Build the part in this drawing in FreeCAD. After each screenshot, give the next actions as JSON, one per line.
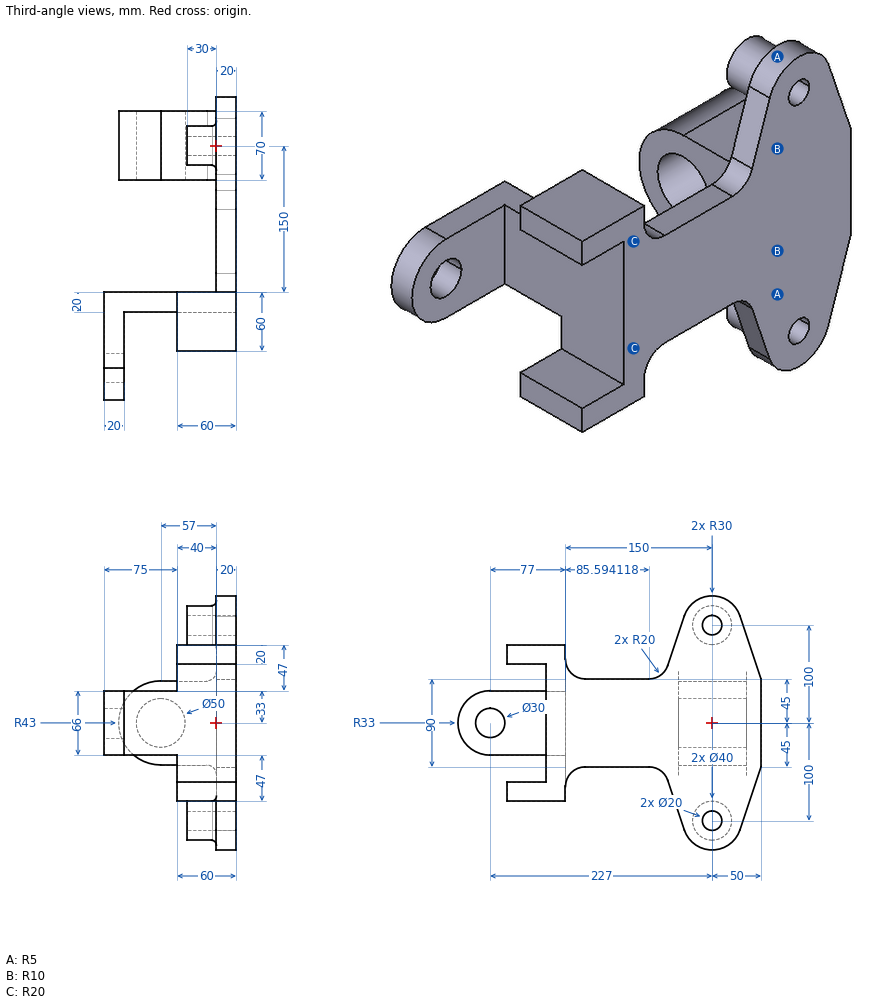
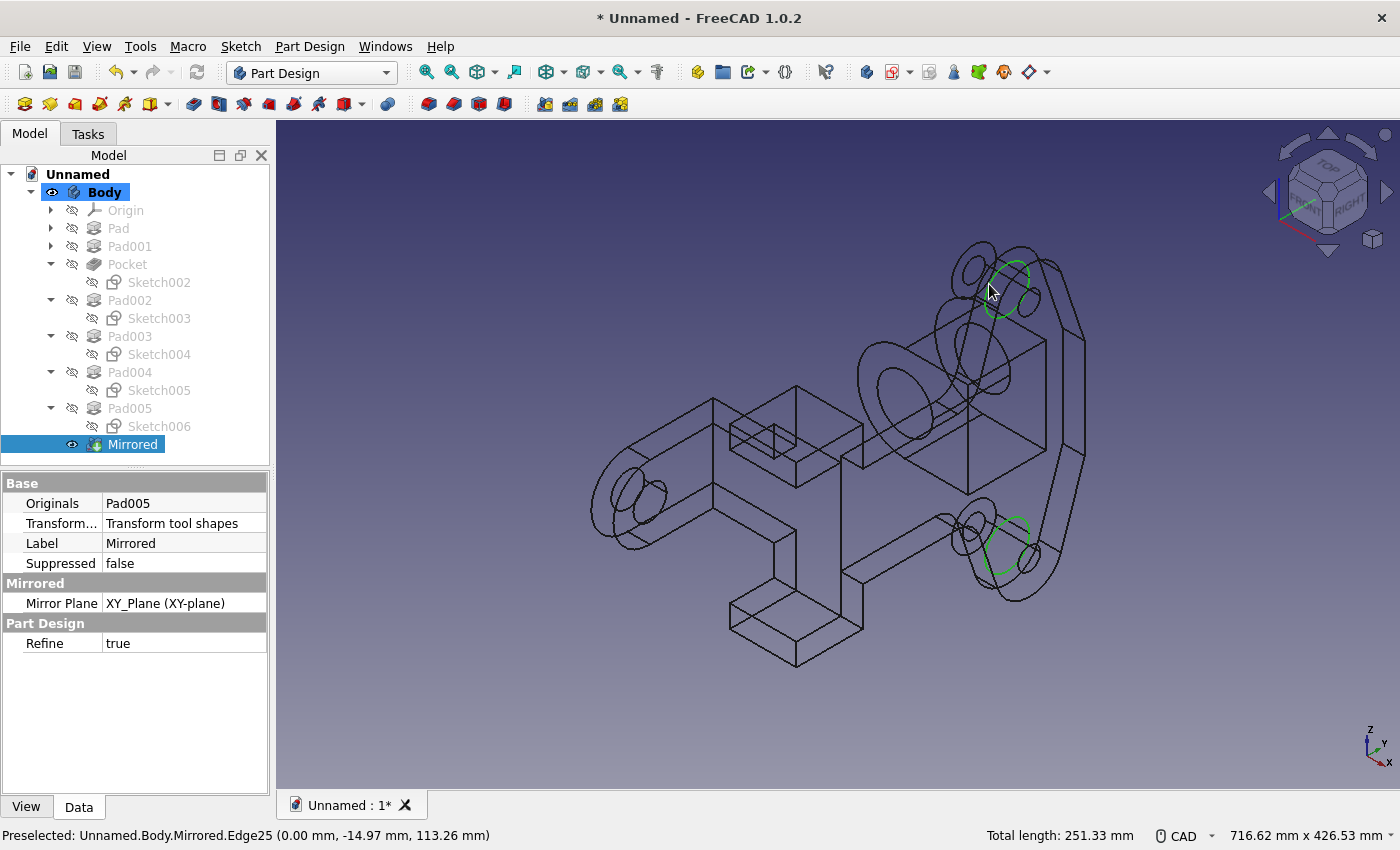
{"action": "key", "text": "v 1"}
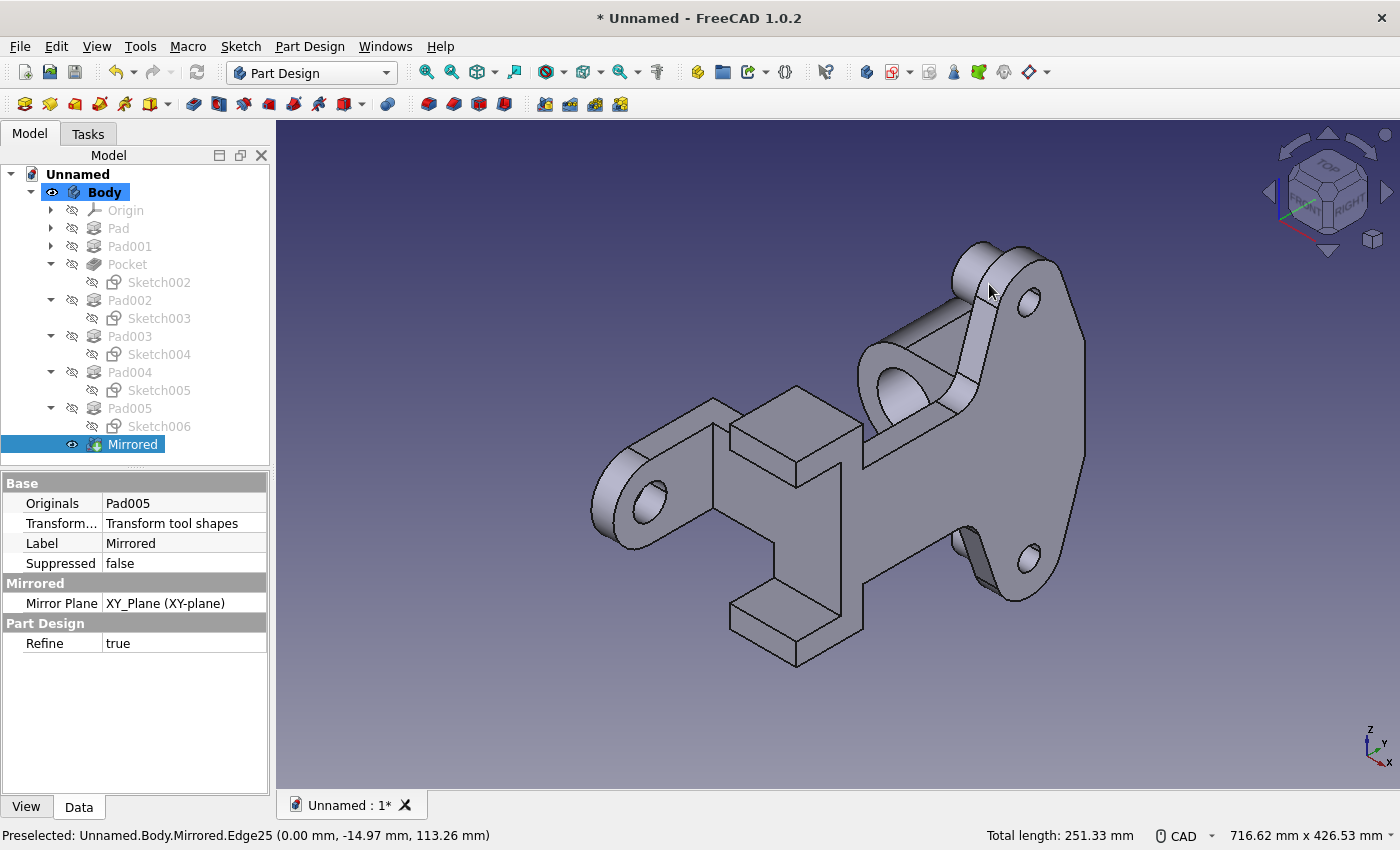
{"action": "left_click", "coordinate": [429, 104]}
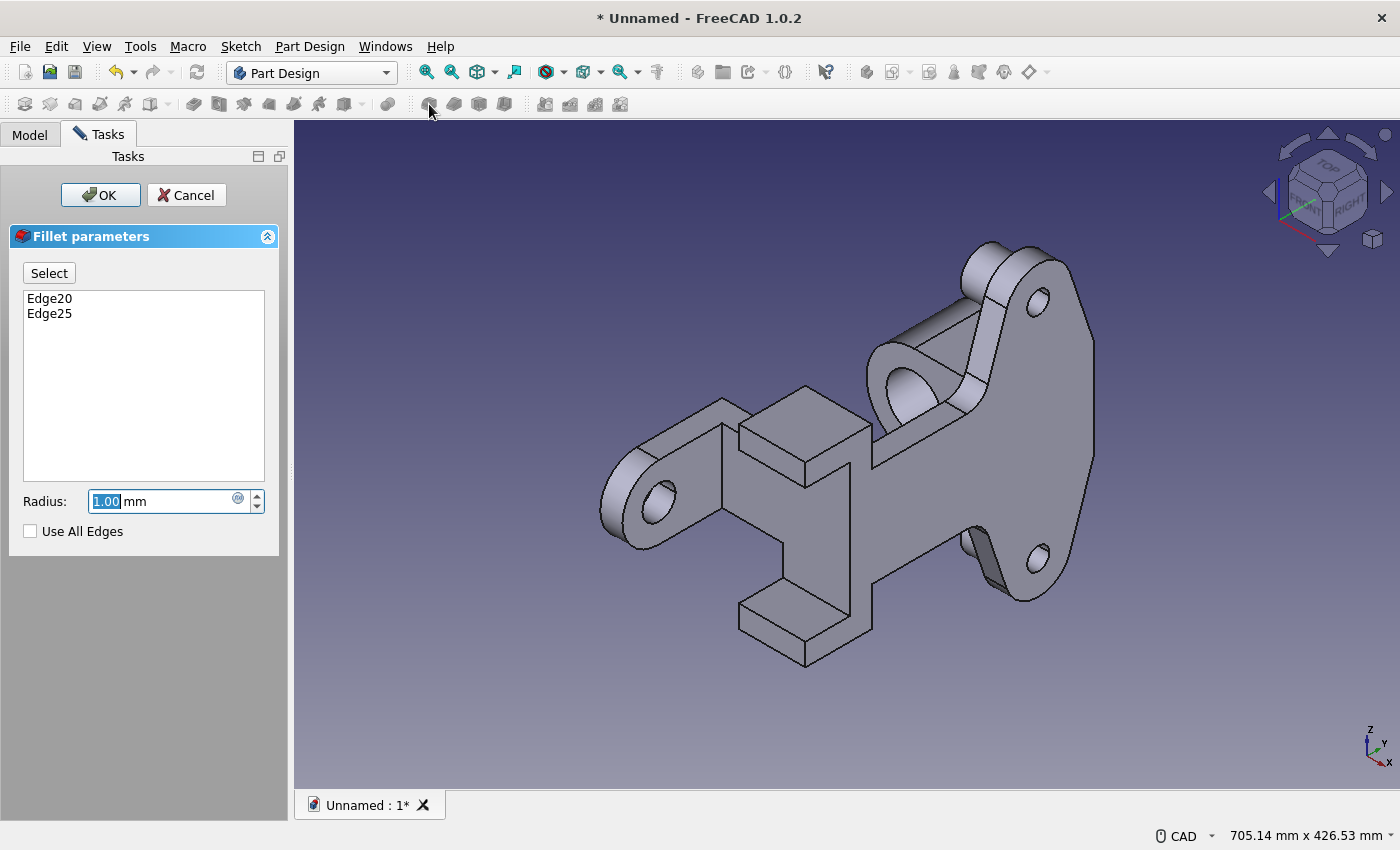
{"action": "type", "text": "5"}
{"action": "key", "text": "Tab"}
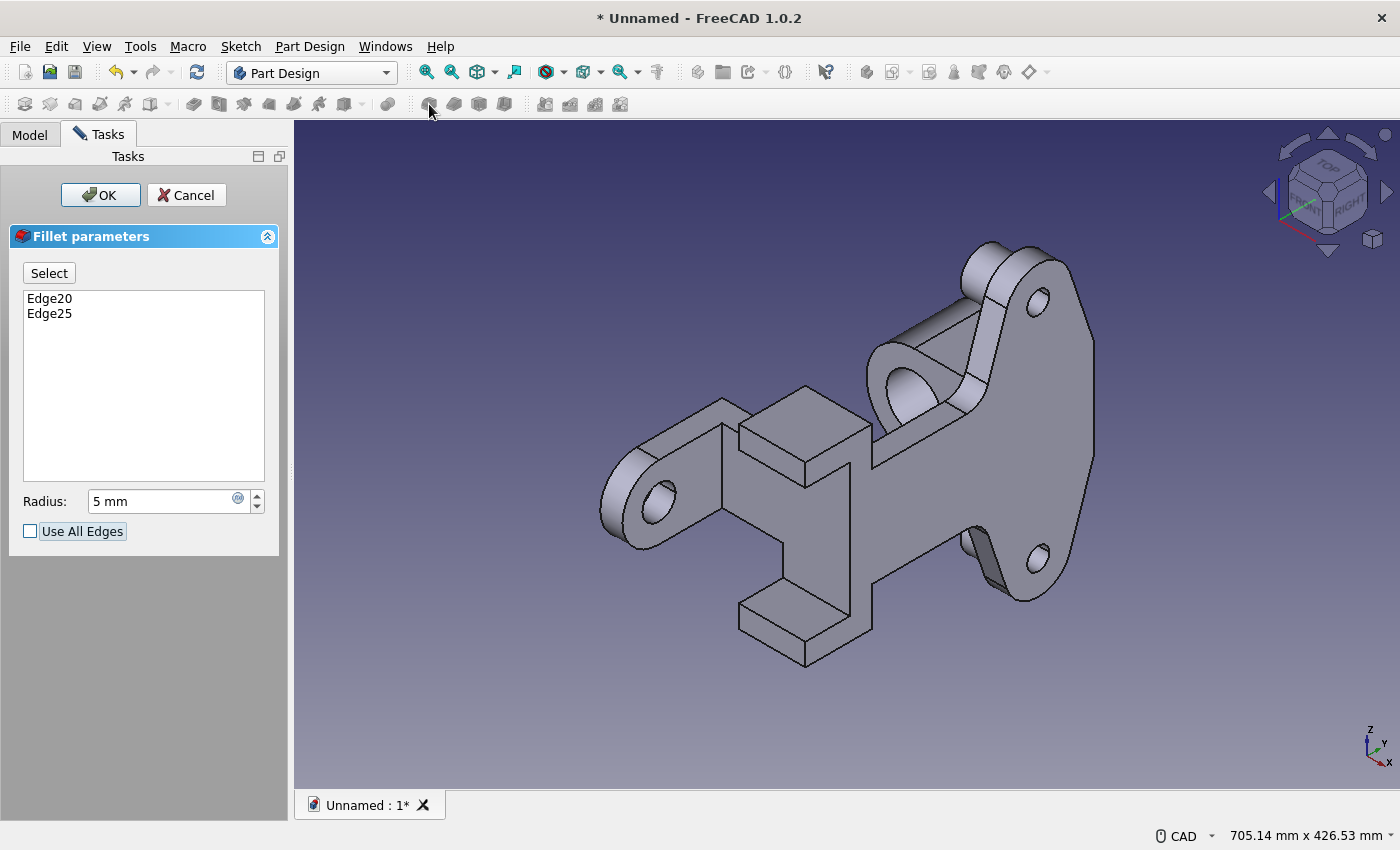
{"action": "left_click", "coordinate": [101, 195]}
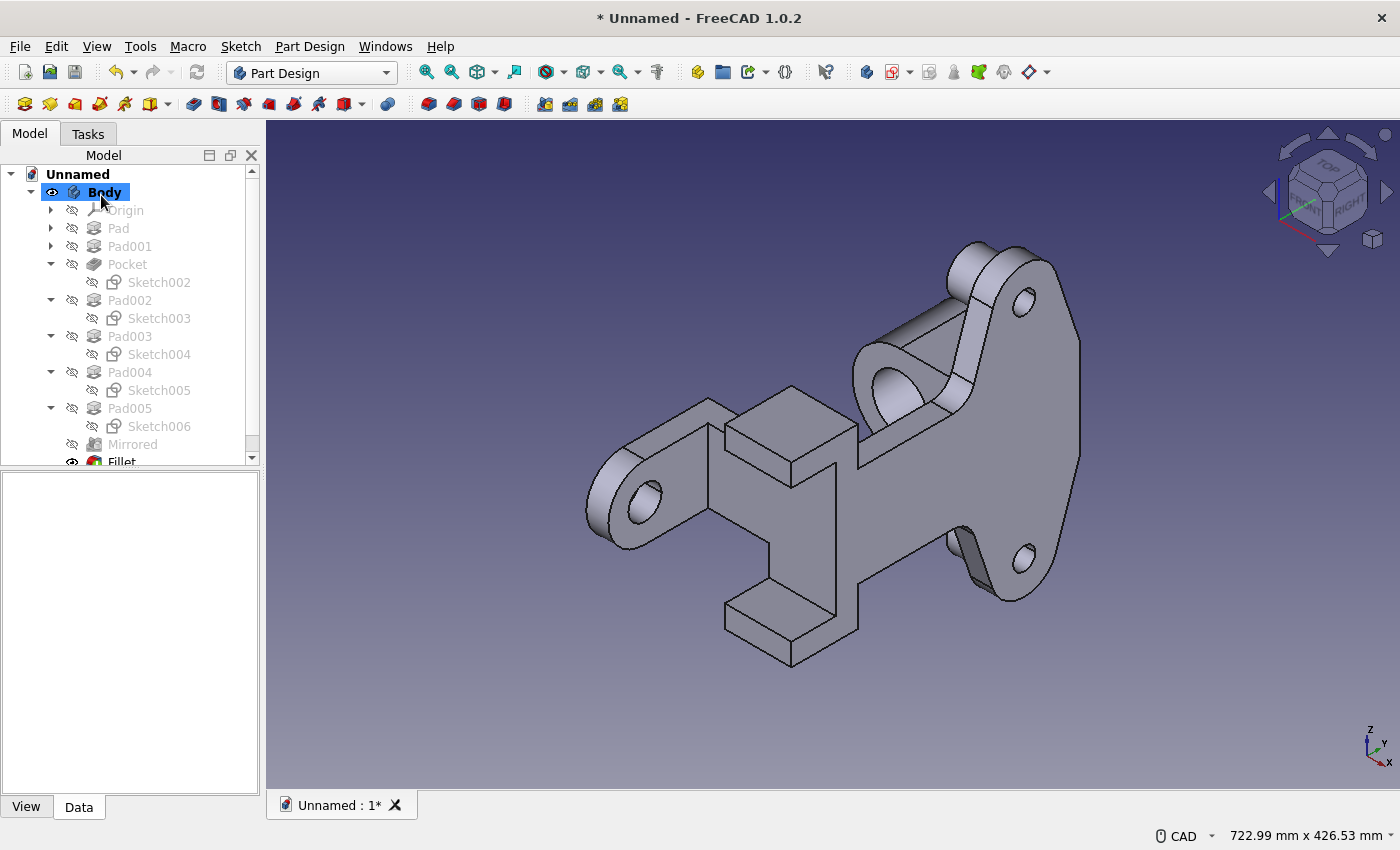
{"action": "key", "text": "2"}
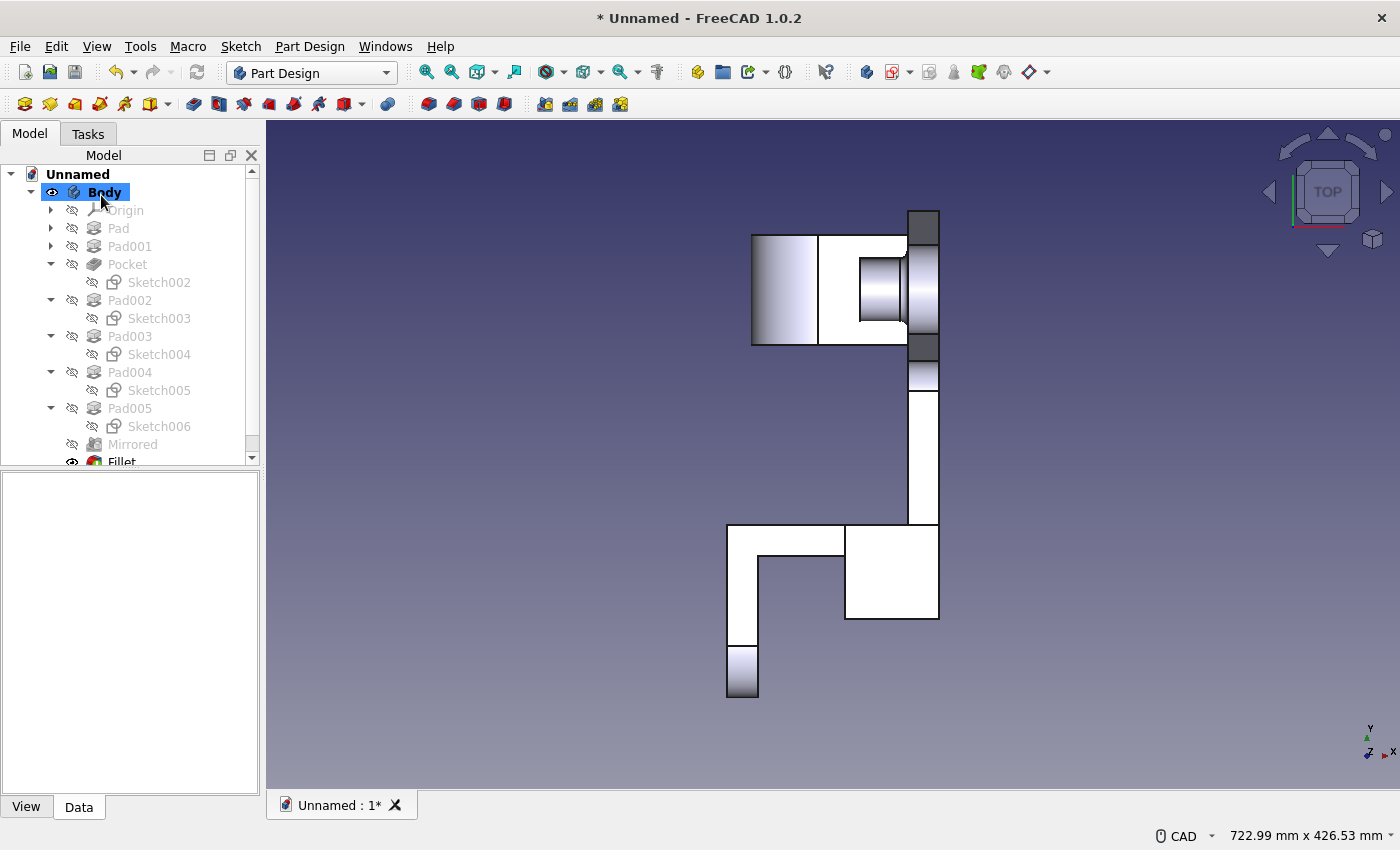
{"action": "key", "text": "0"}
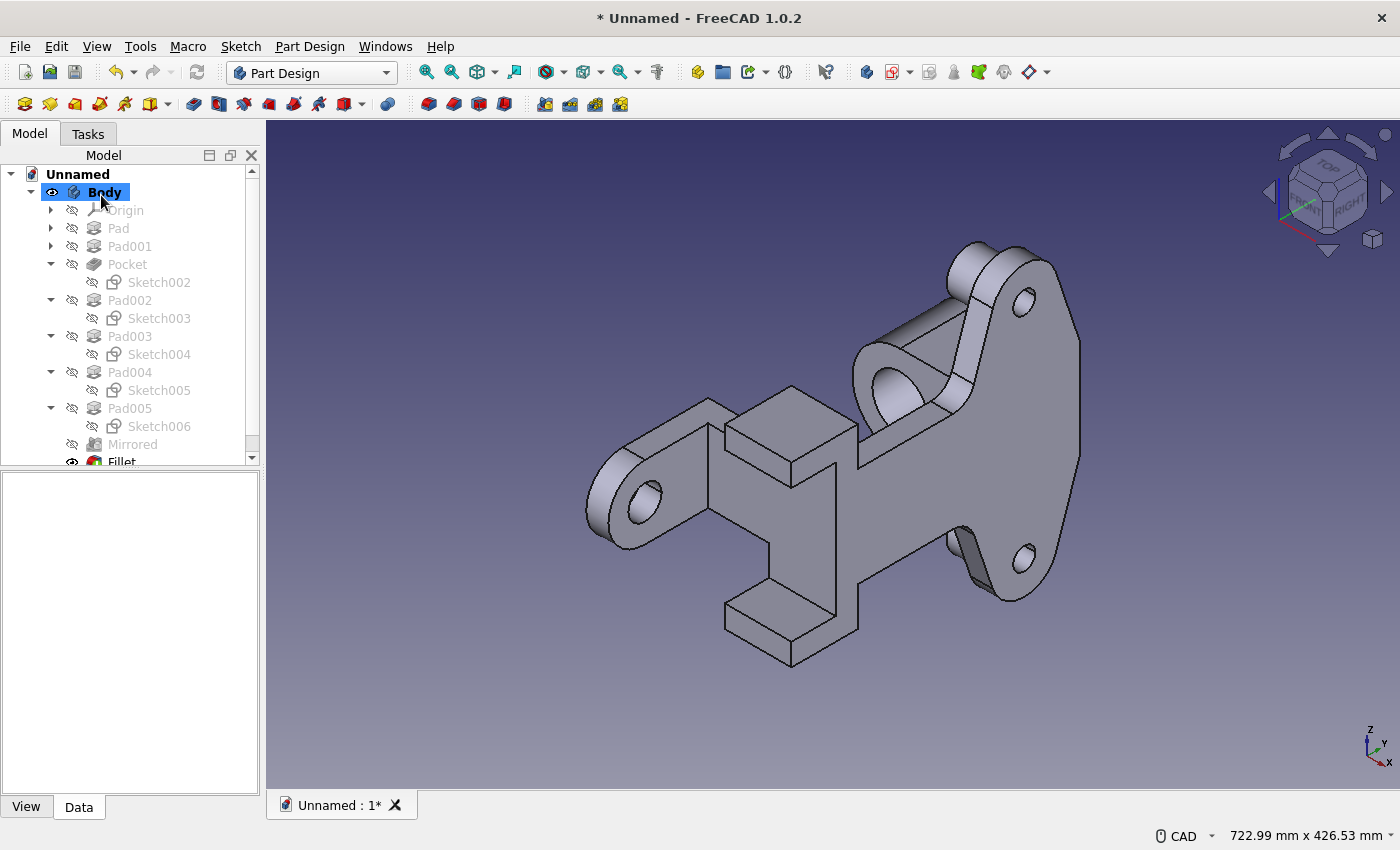
{"action": "key", "text": "1"}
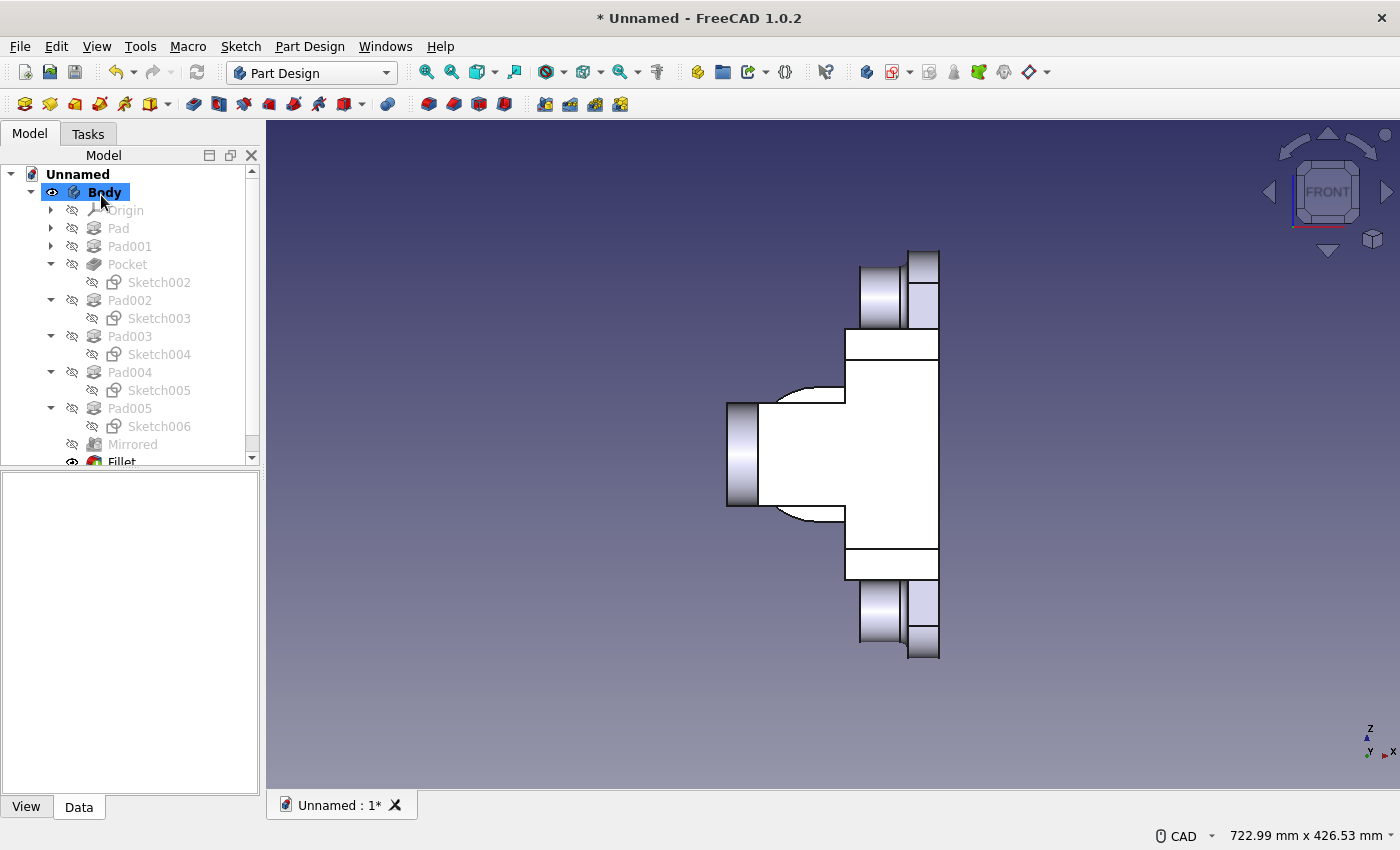
{"action": "key", "text": "3"}